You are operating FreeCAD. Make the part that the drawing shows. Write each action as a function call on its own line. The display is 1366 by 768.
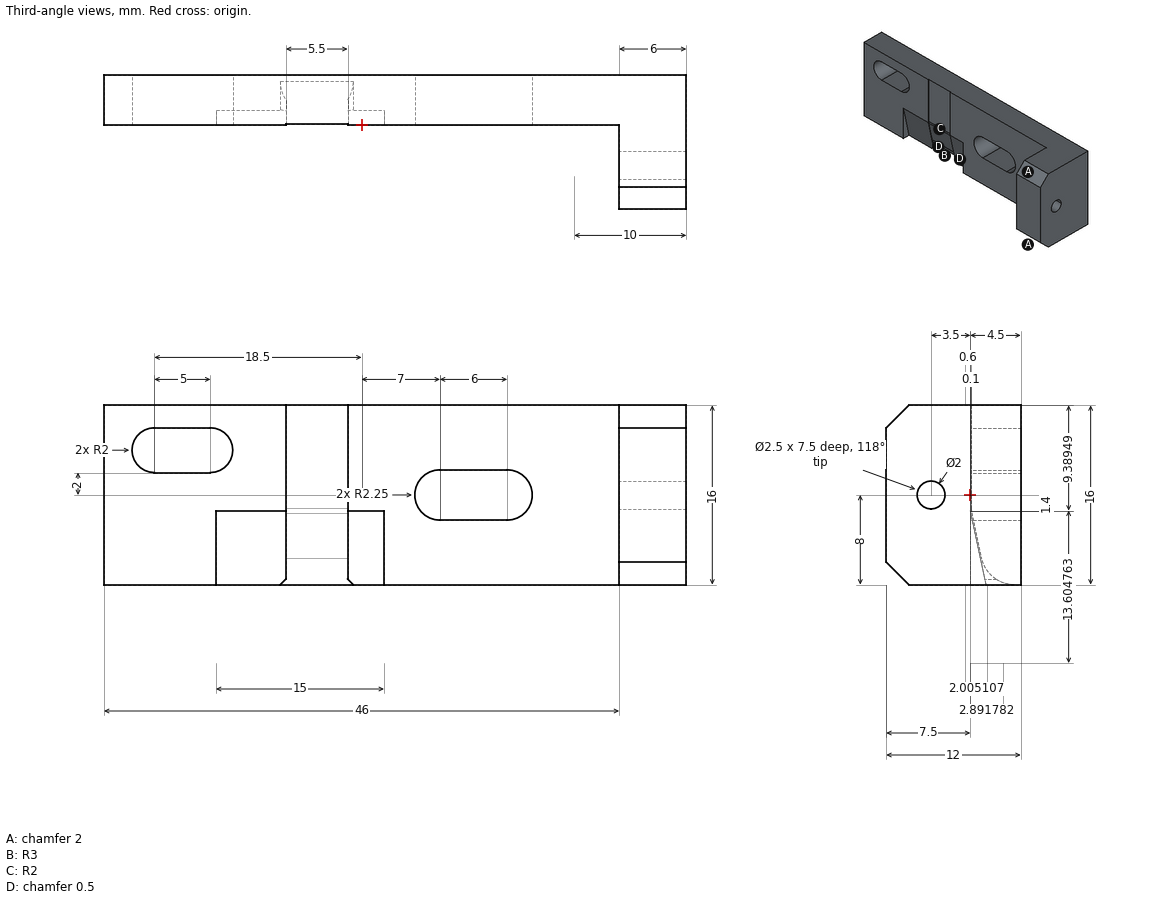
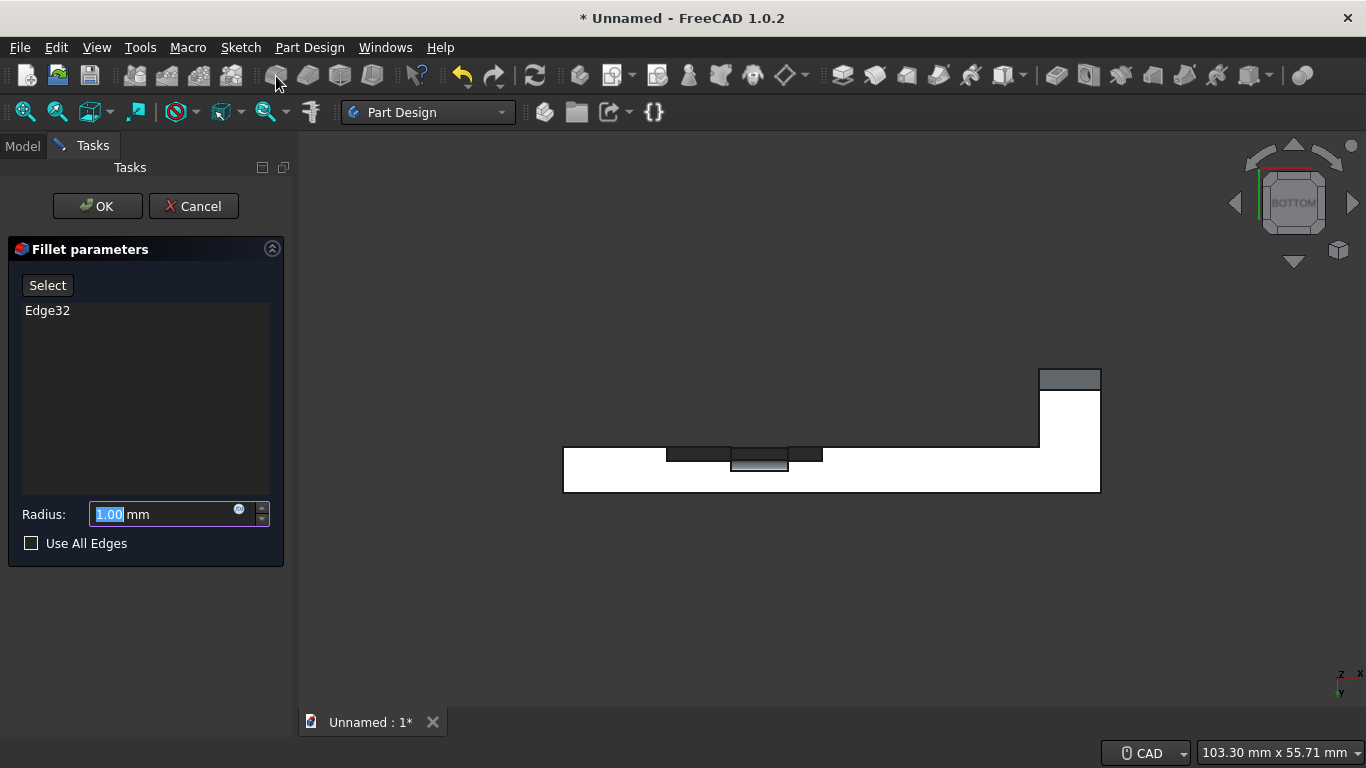
text(3)
key(Tab)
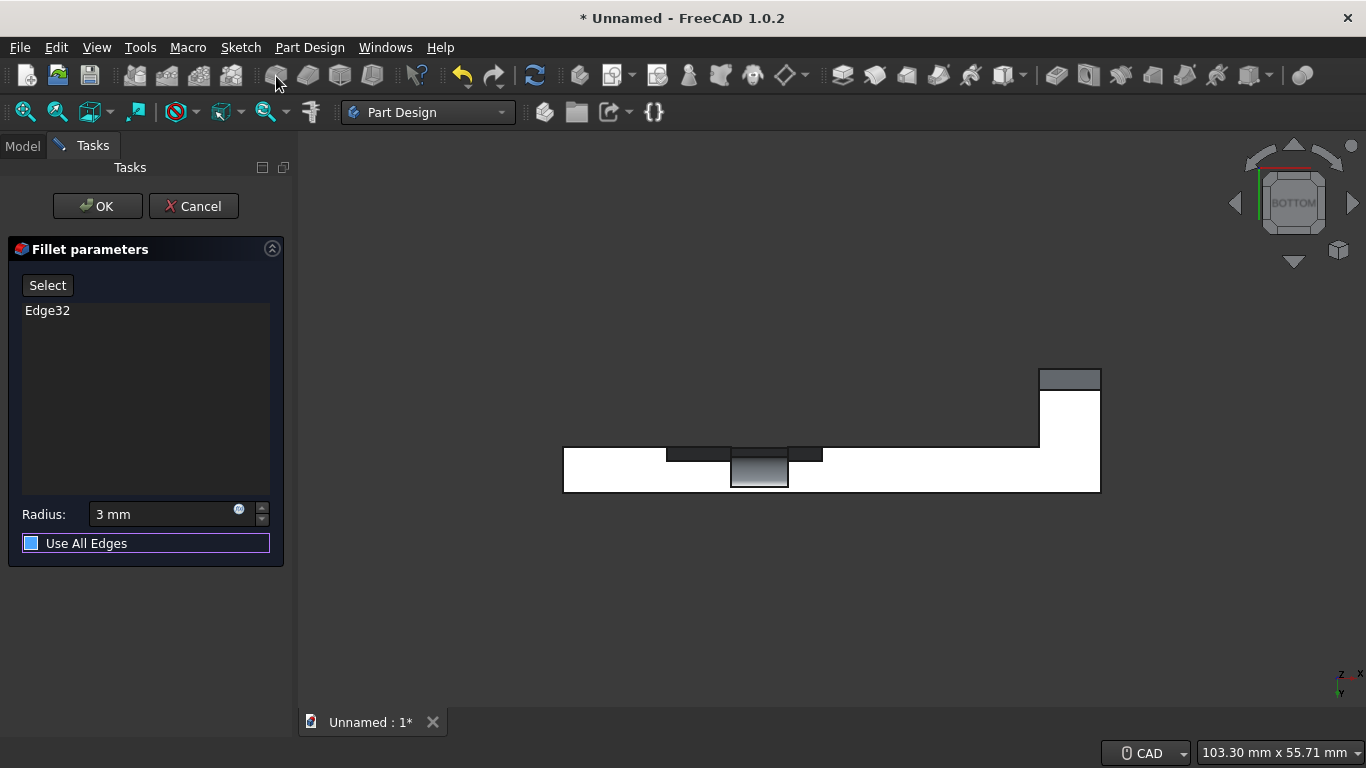
click(98, 206)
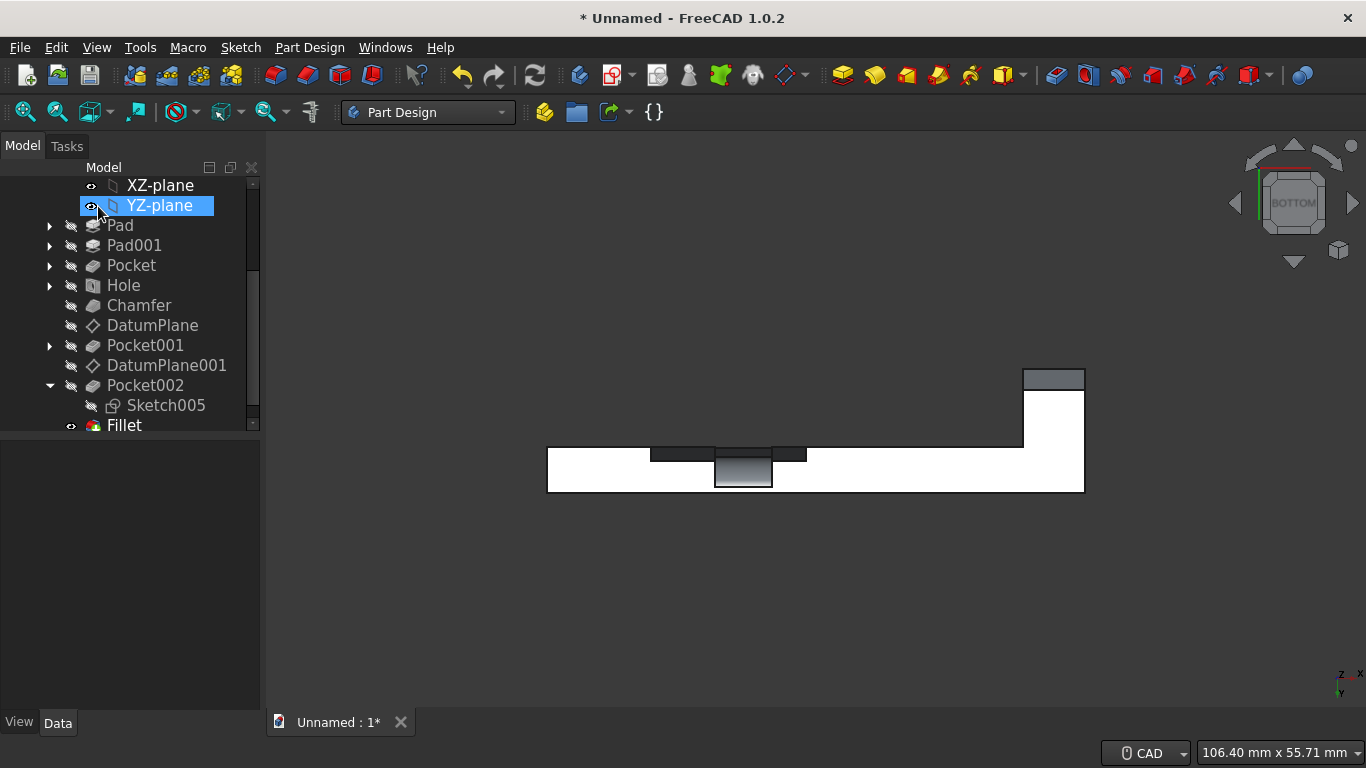
key(0)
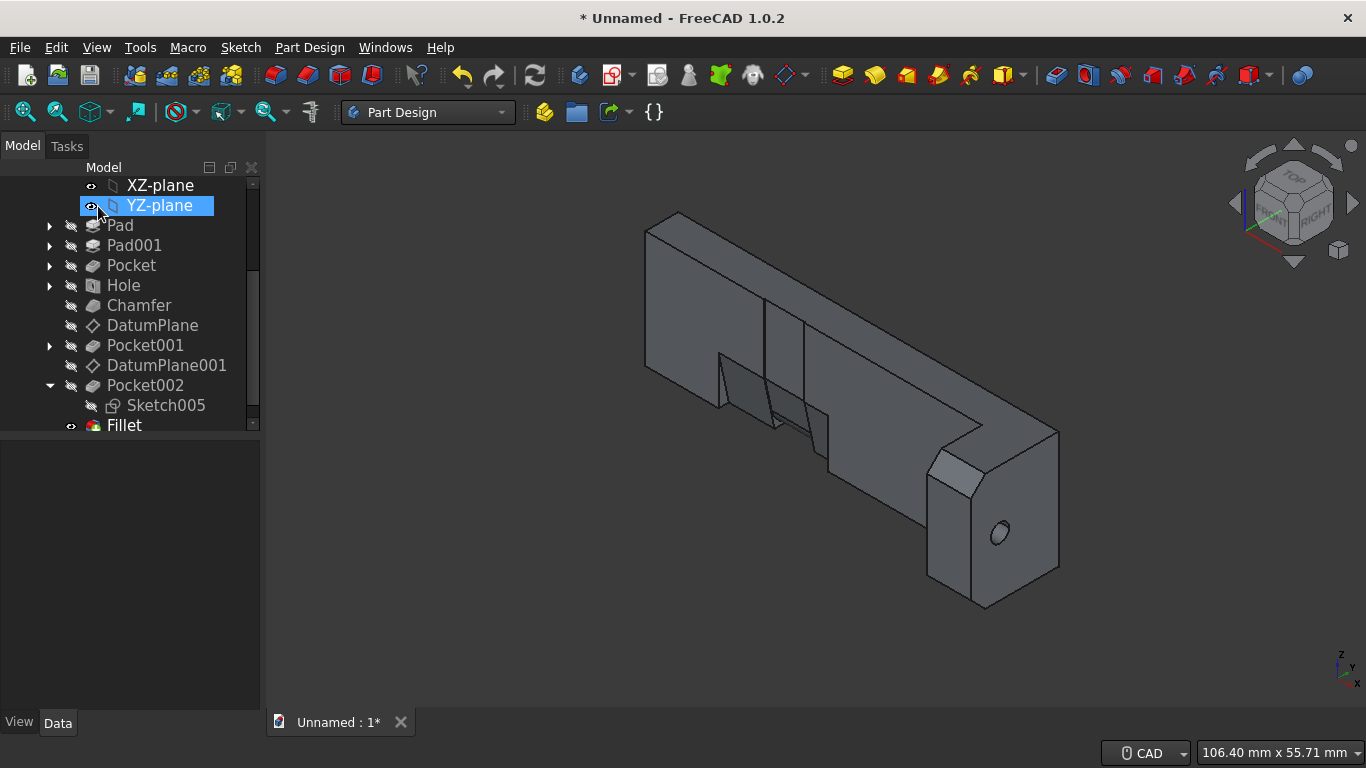
key(2)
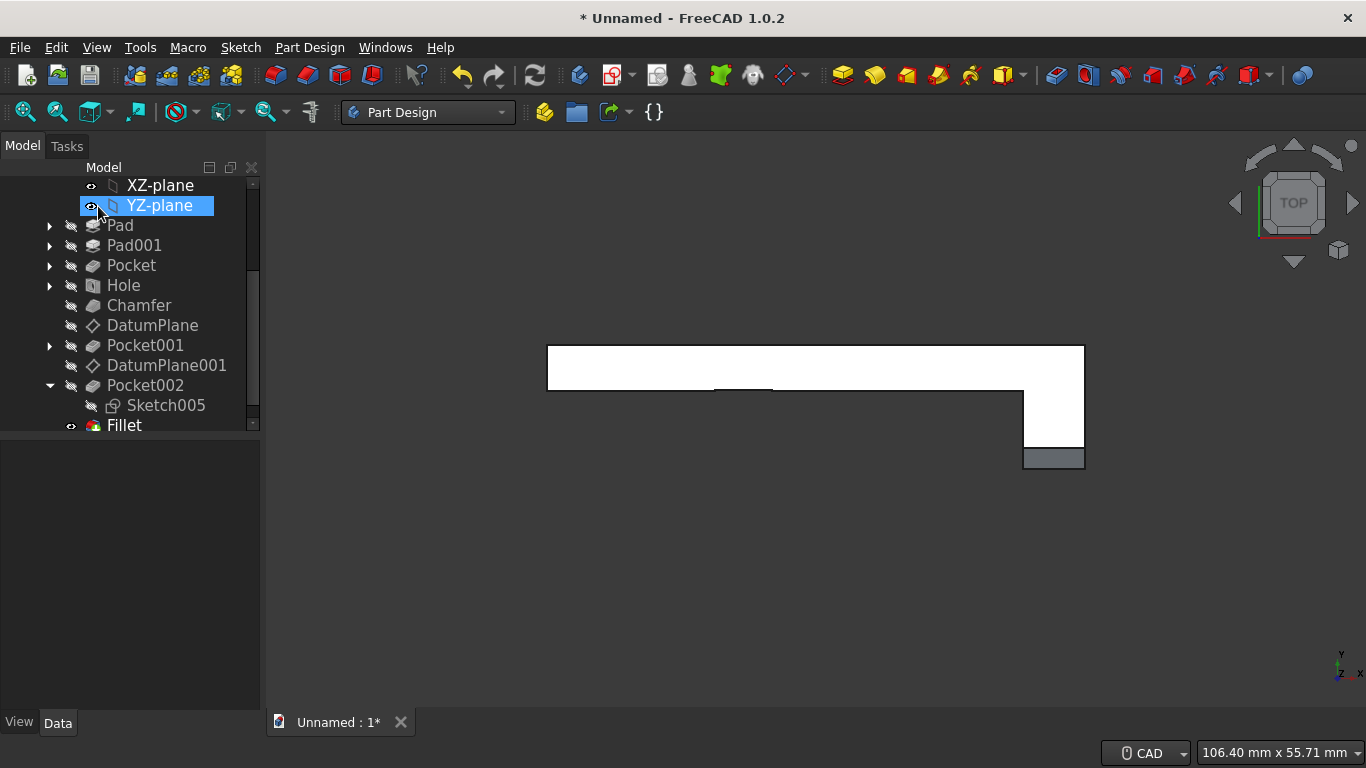
key(1)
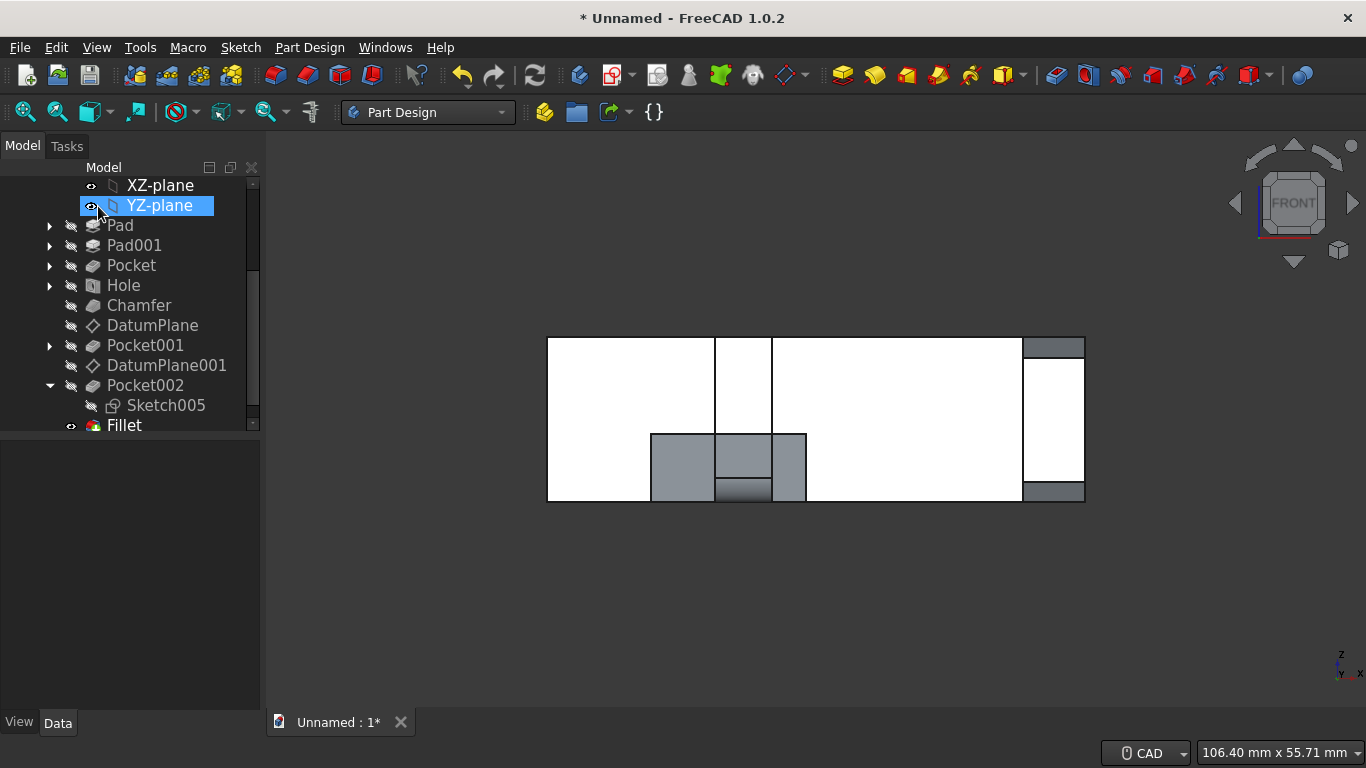
key(3)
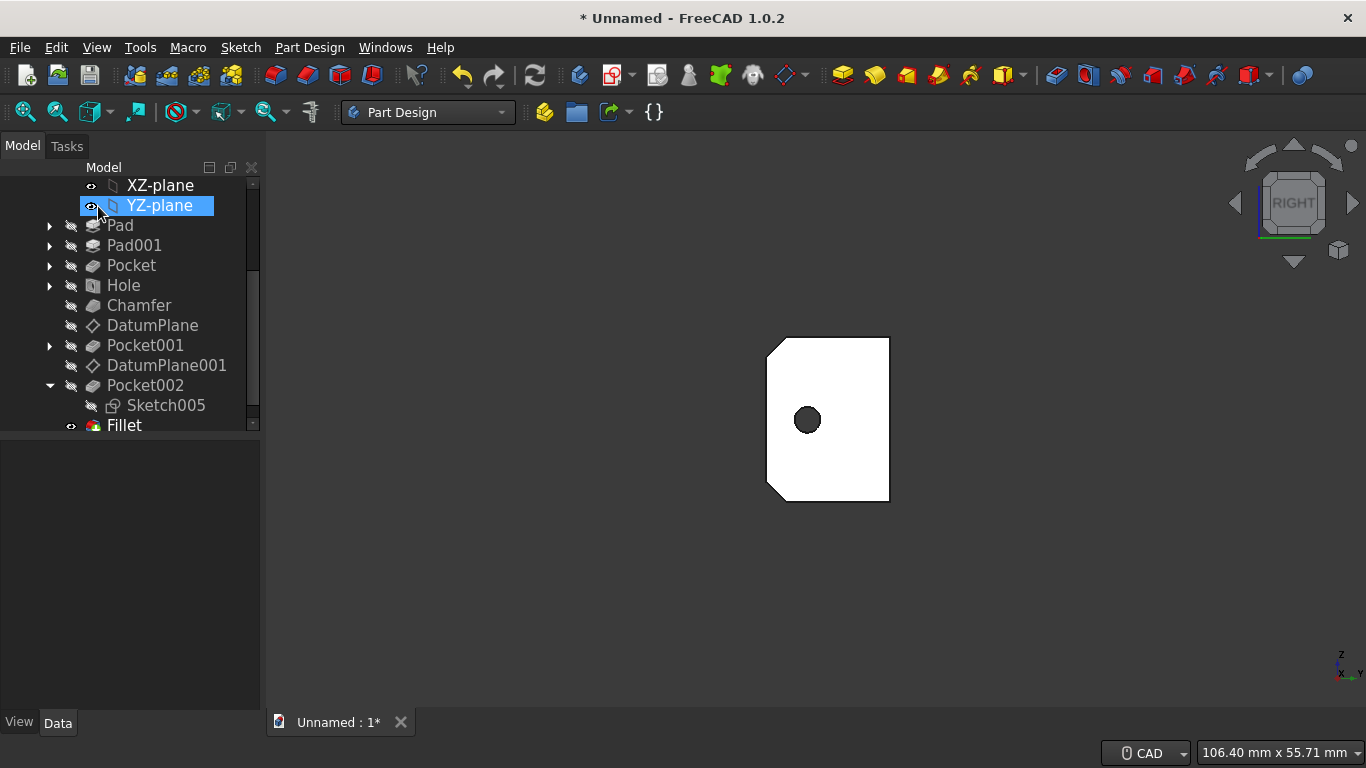
click(26, 112)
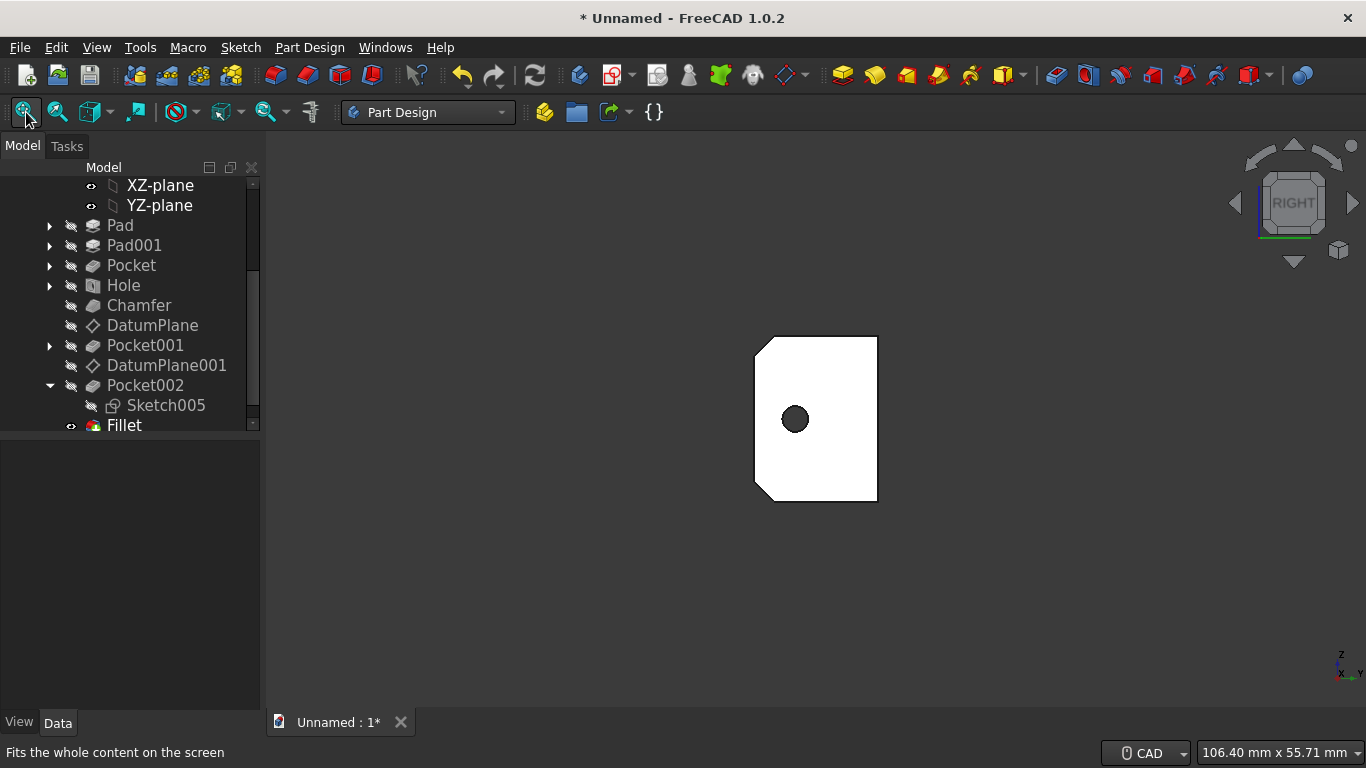
key(5)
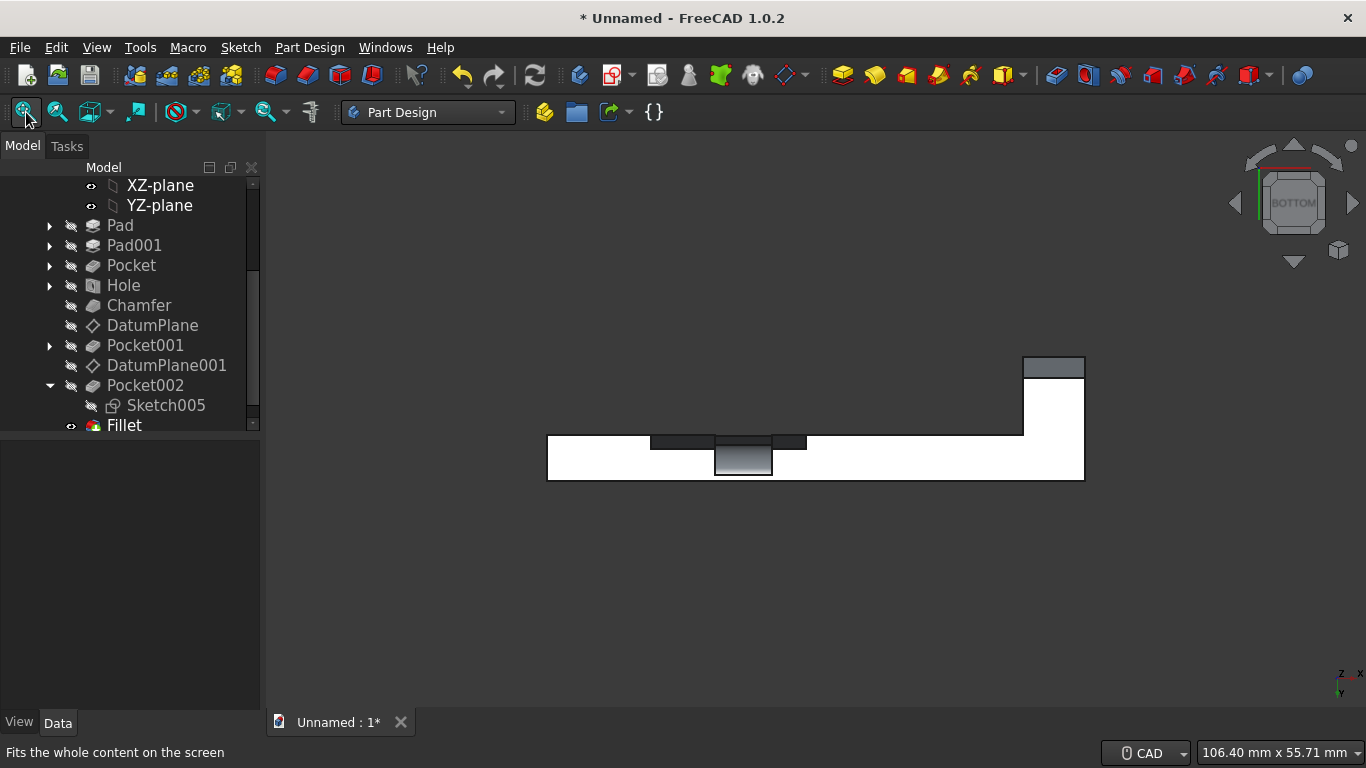
key(4)